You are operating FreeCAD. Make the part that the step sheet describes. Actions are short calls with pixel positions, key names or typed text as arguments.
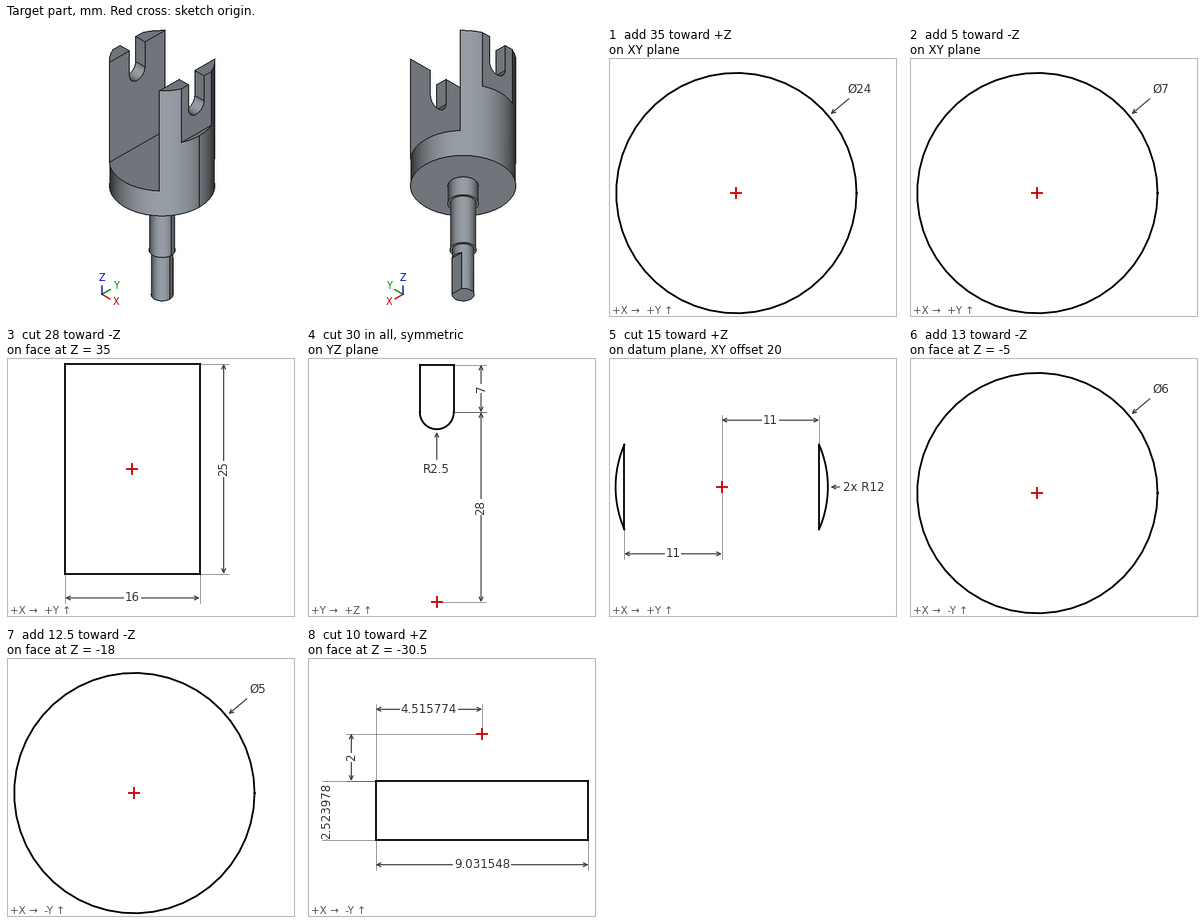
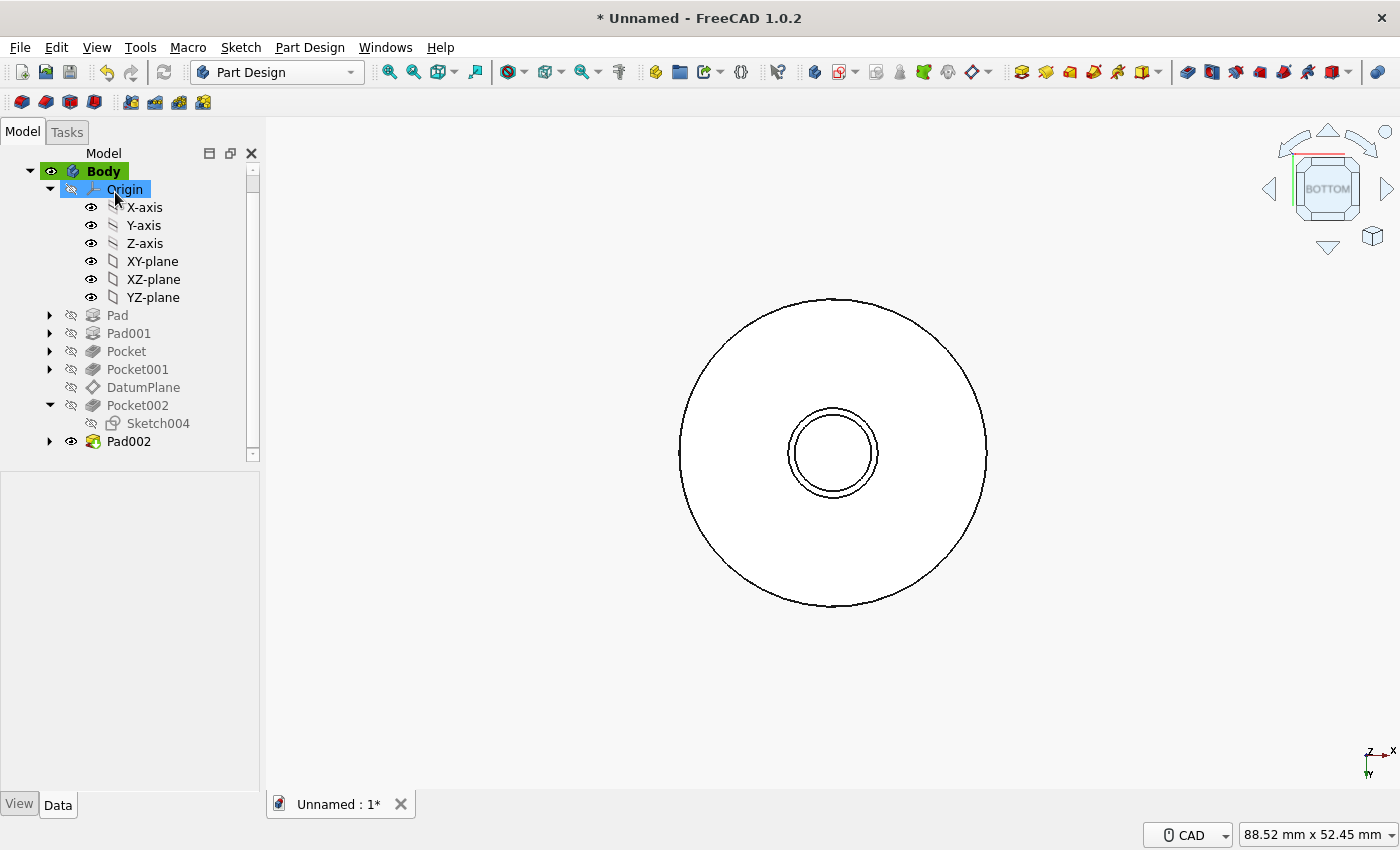
click(833, 452)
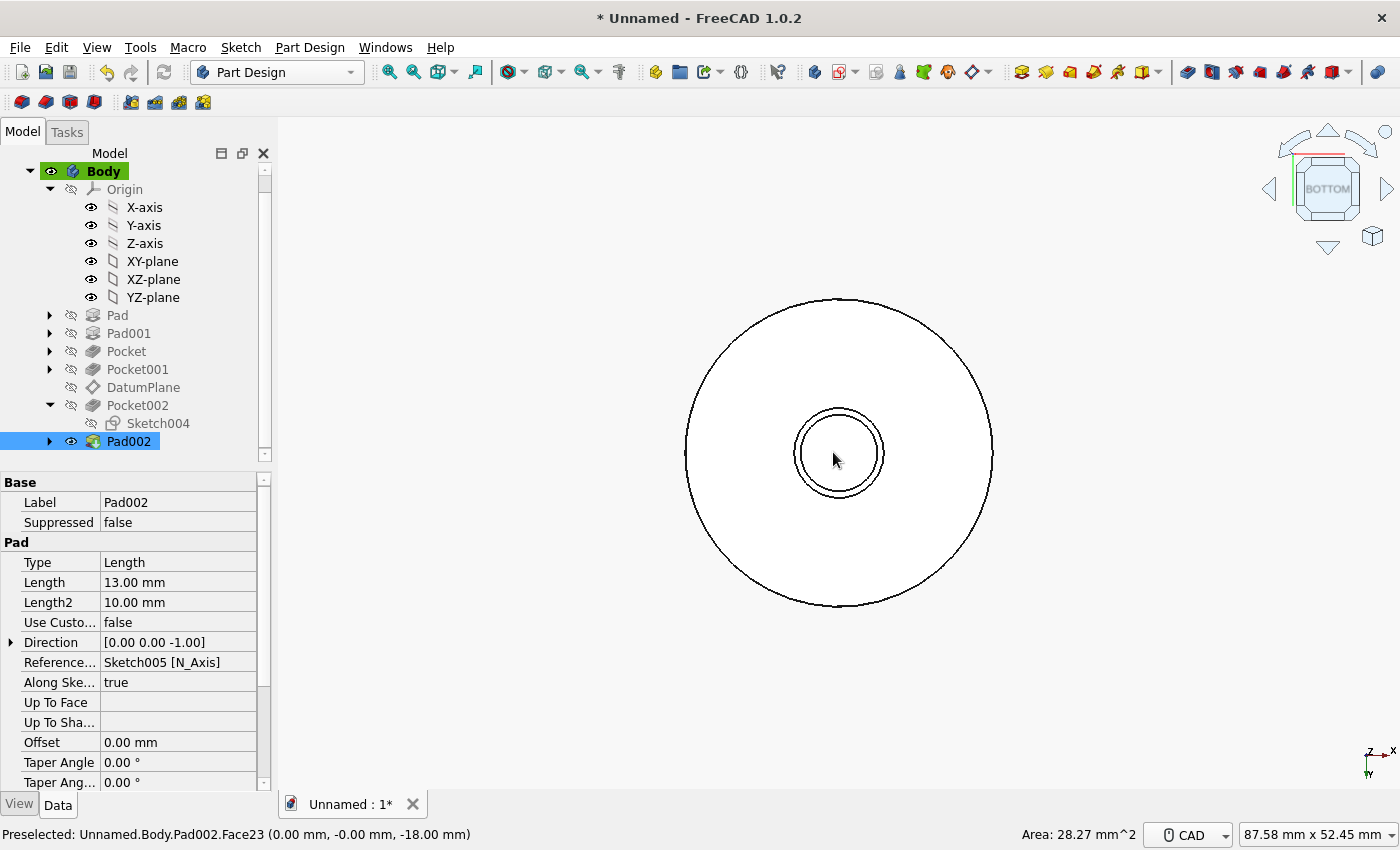
click(840, 72)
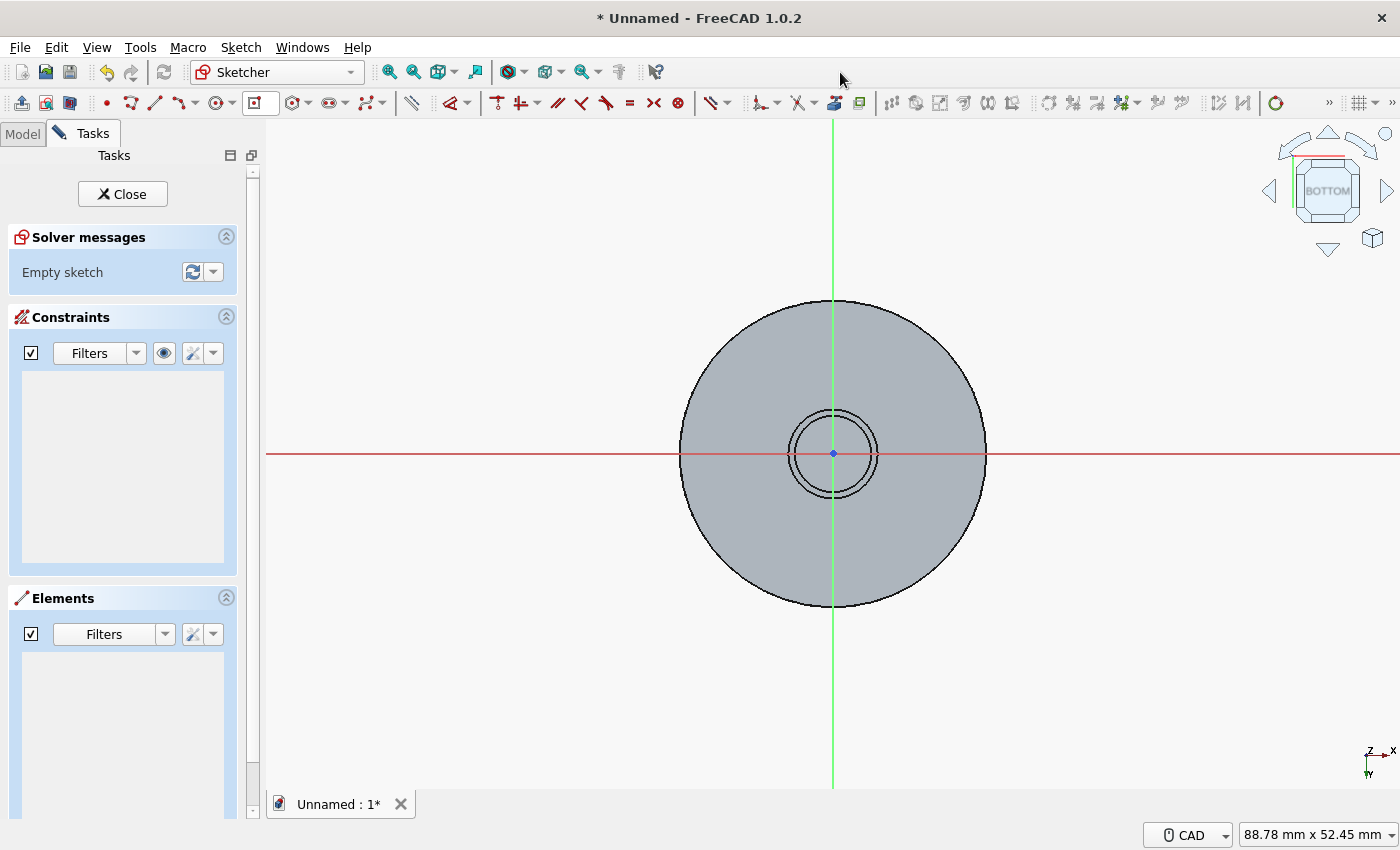
scroll(844, 454, up, 10)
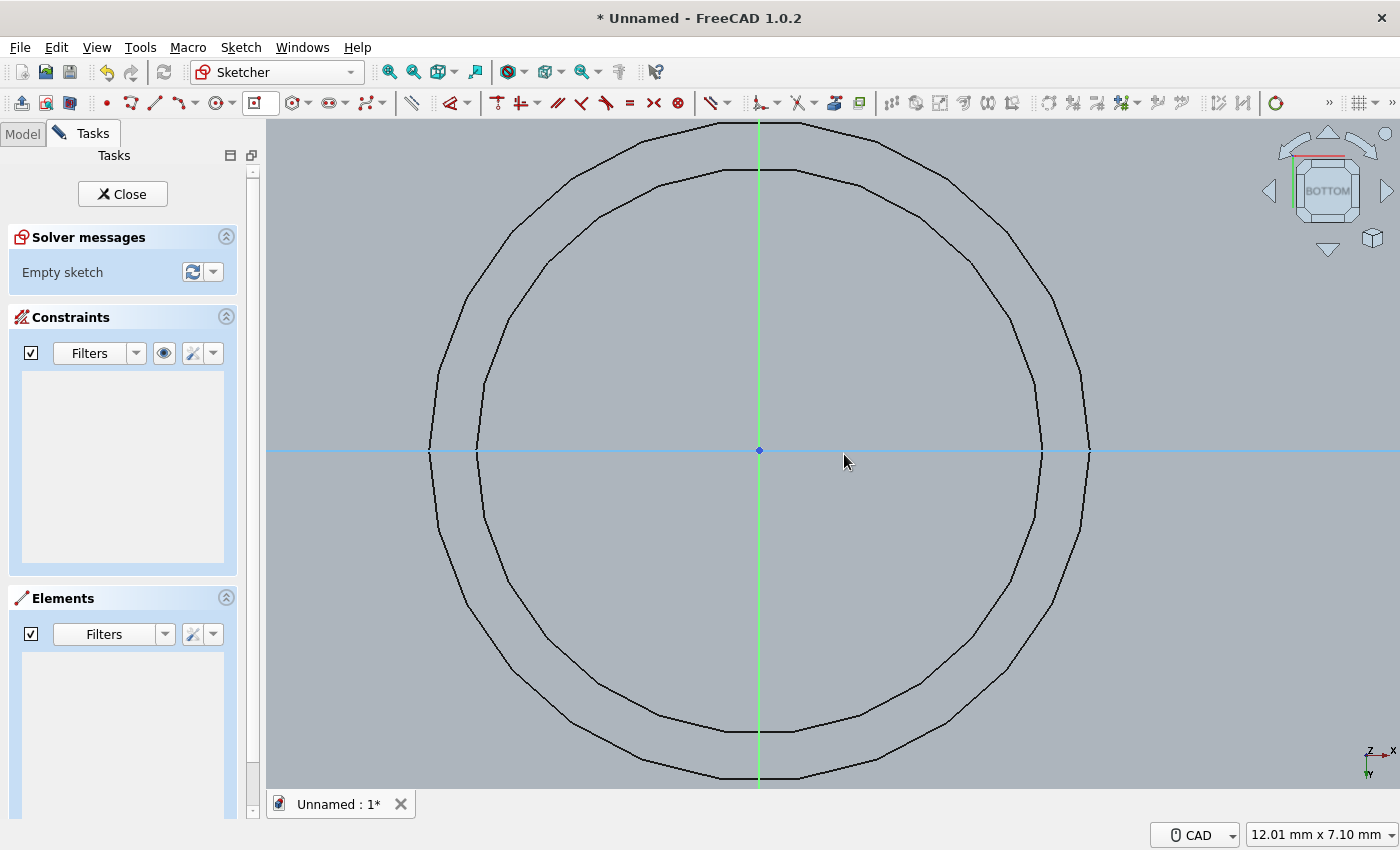
key(g)
key(c)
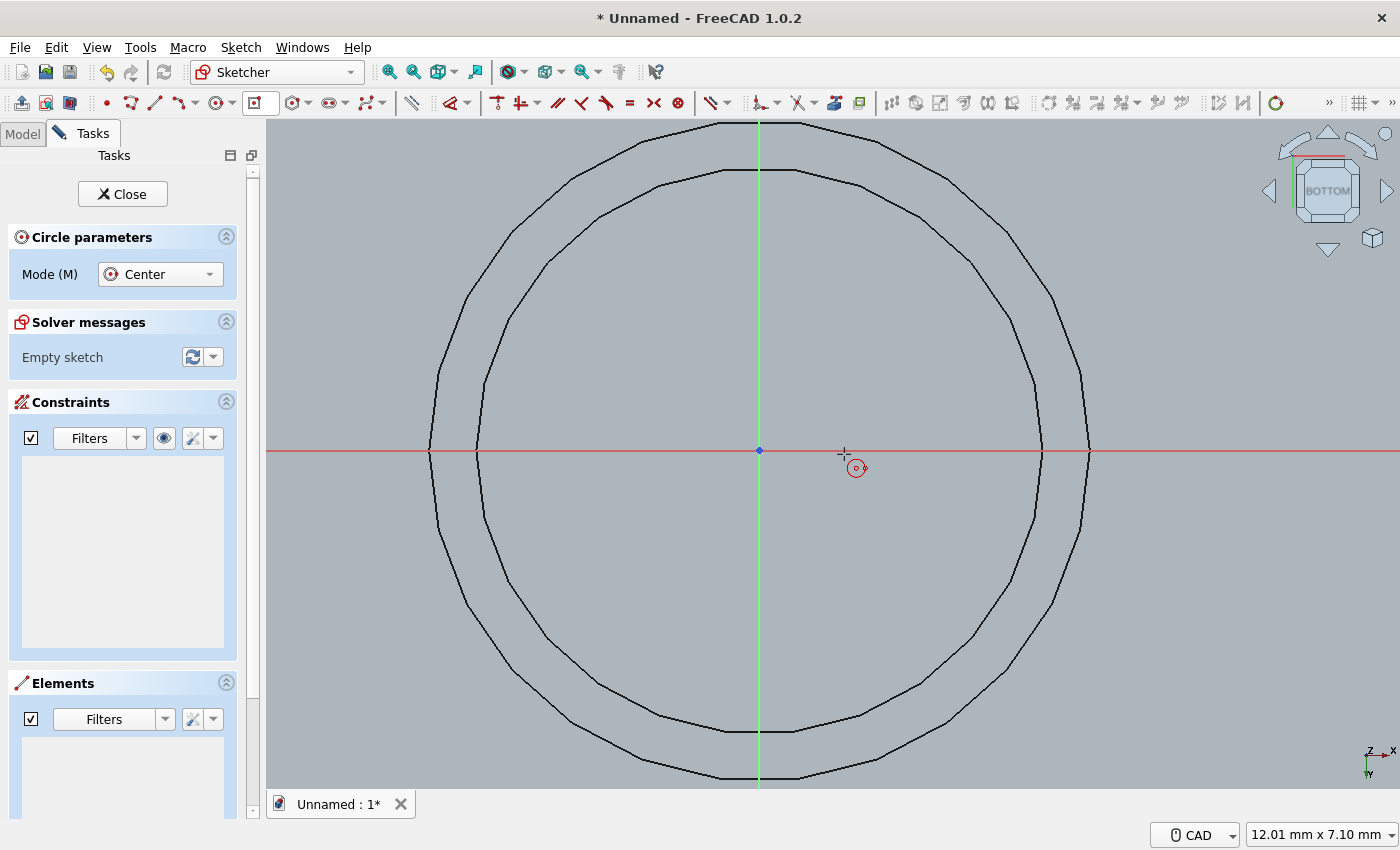
click(759, 451)
click(926, 284)
key(Escape)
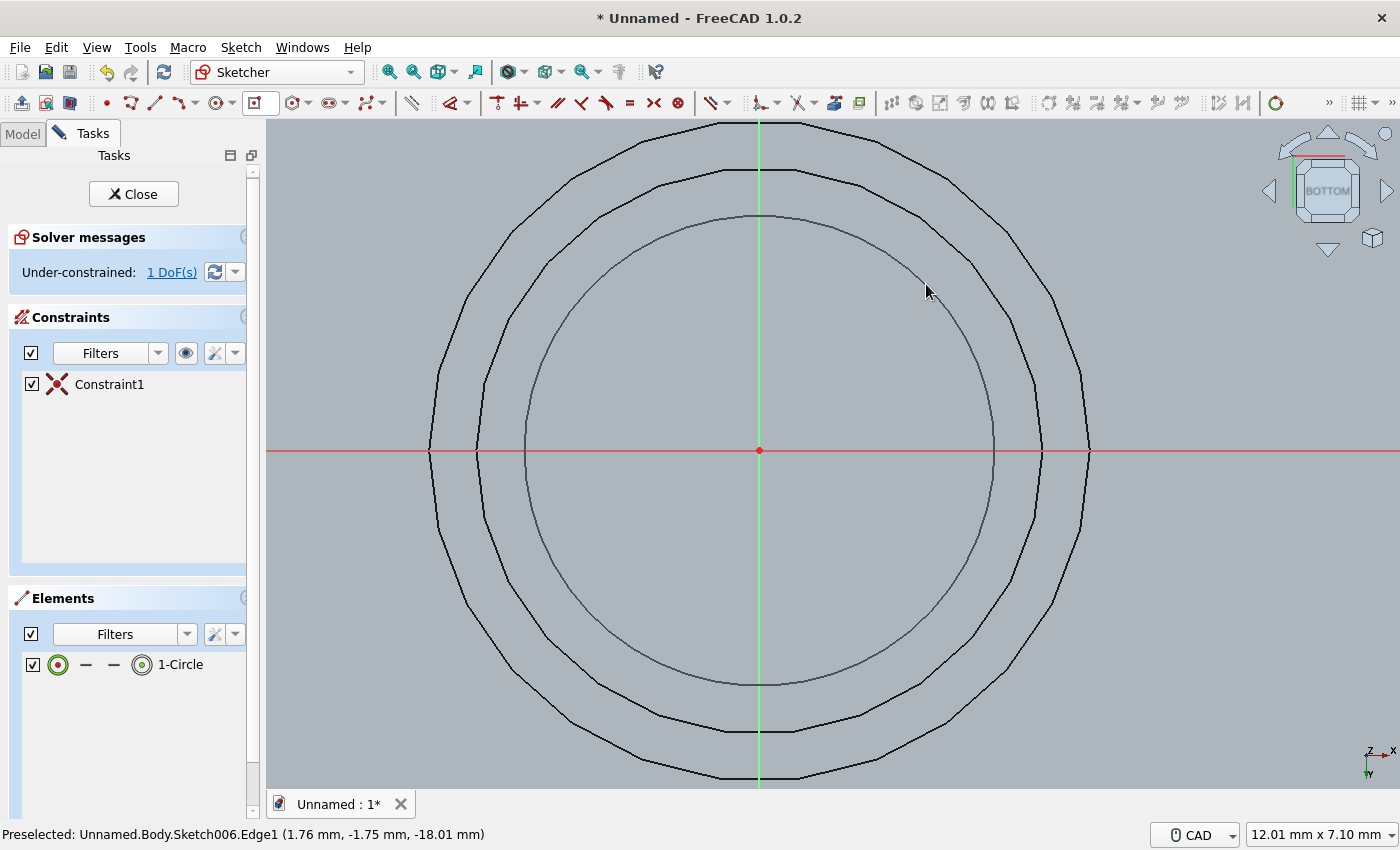
click(450, 104)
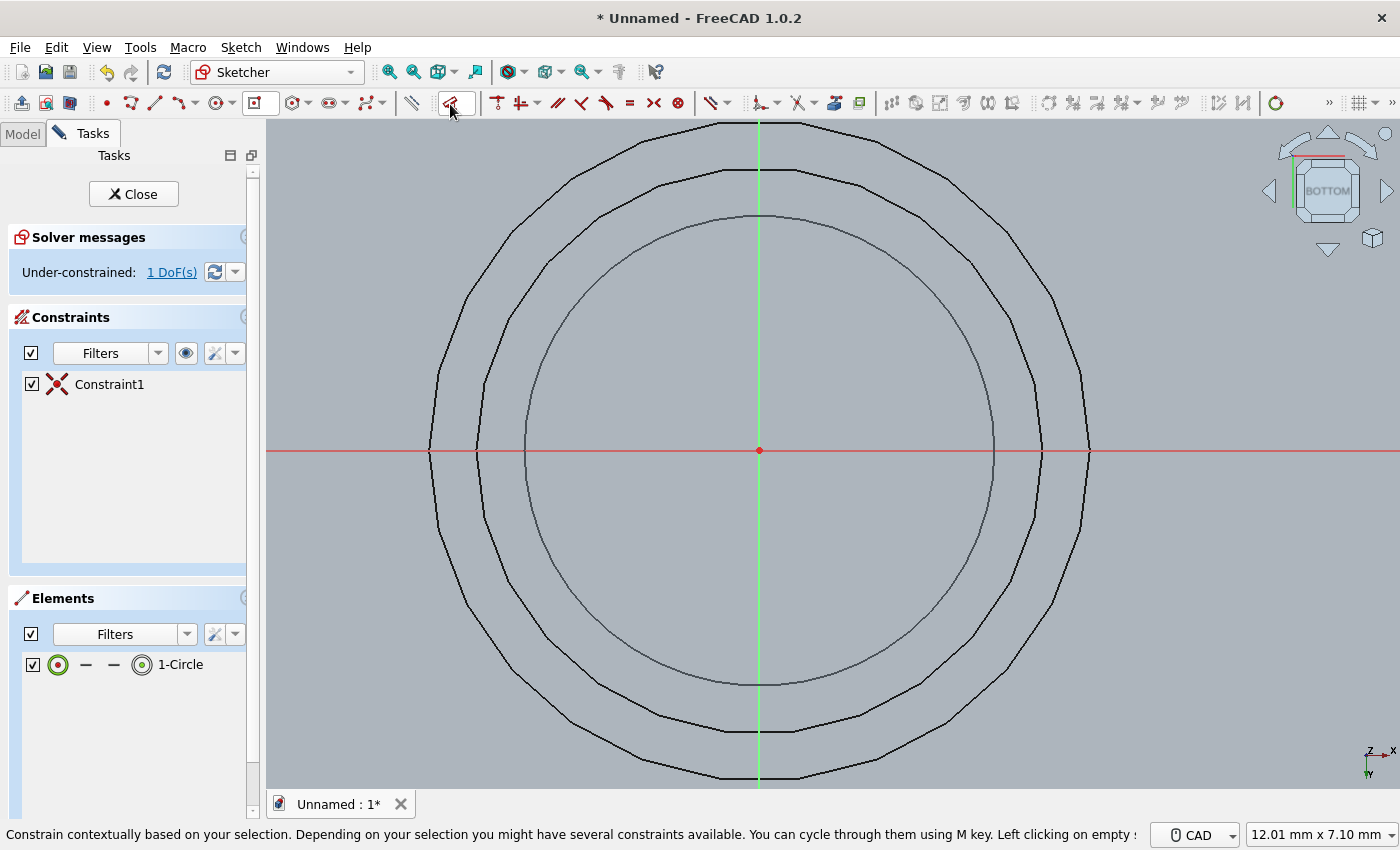
click(925, 284)
click(948, 261)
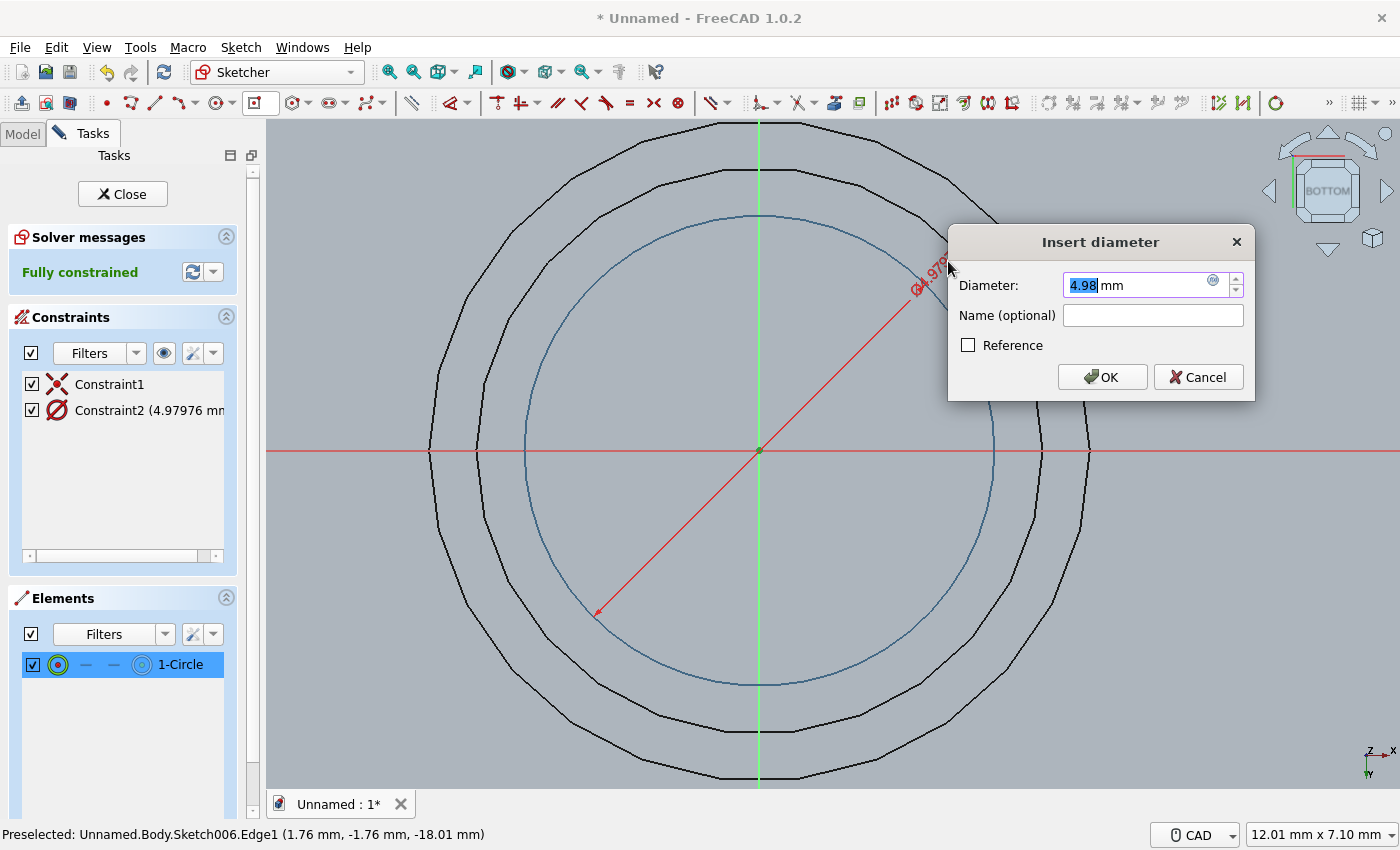
text(5)
key(Return)
key(Escape)